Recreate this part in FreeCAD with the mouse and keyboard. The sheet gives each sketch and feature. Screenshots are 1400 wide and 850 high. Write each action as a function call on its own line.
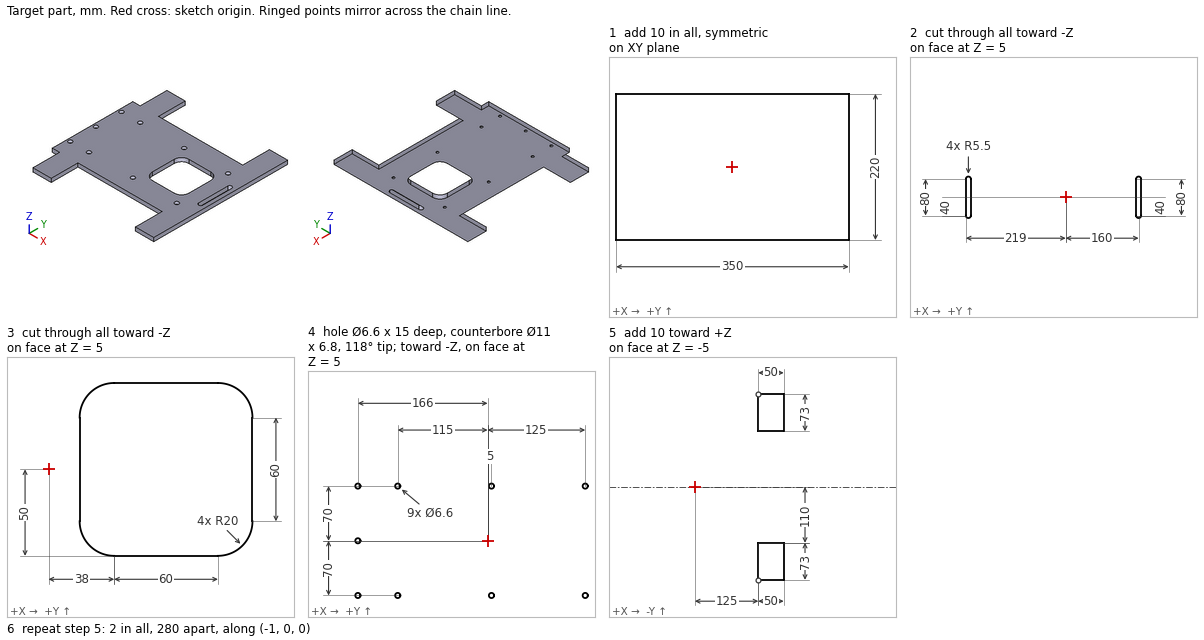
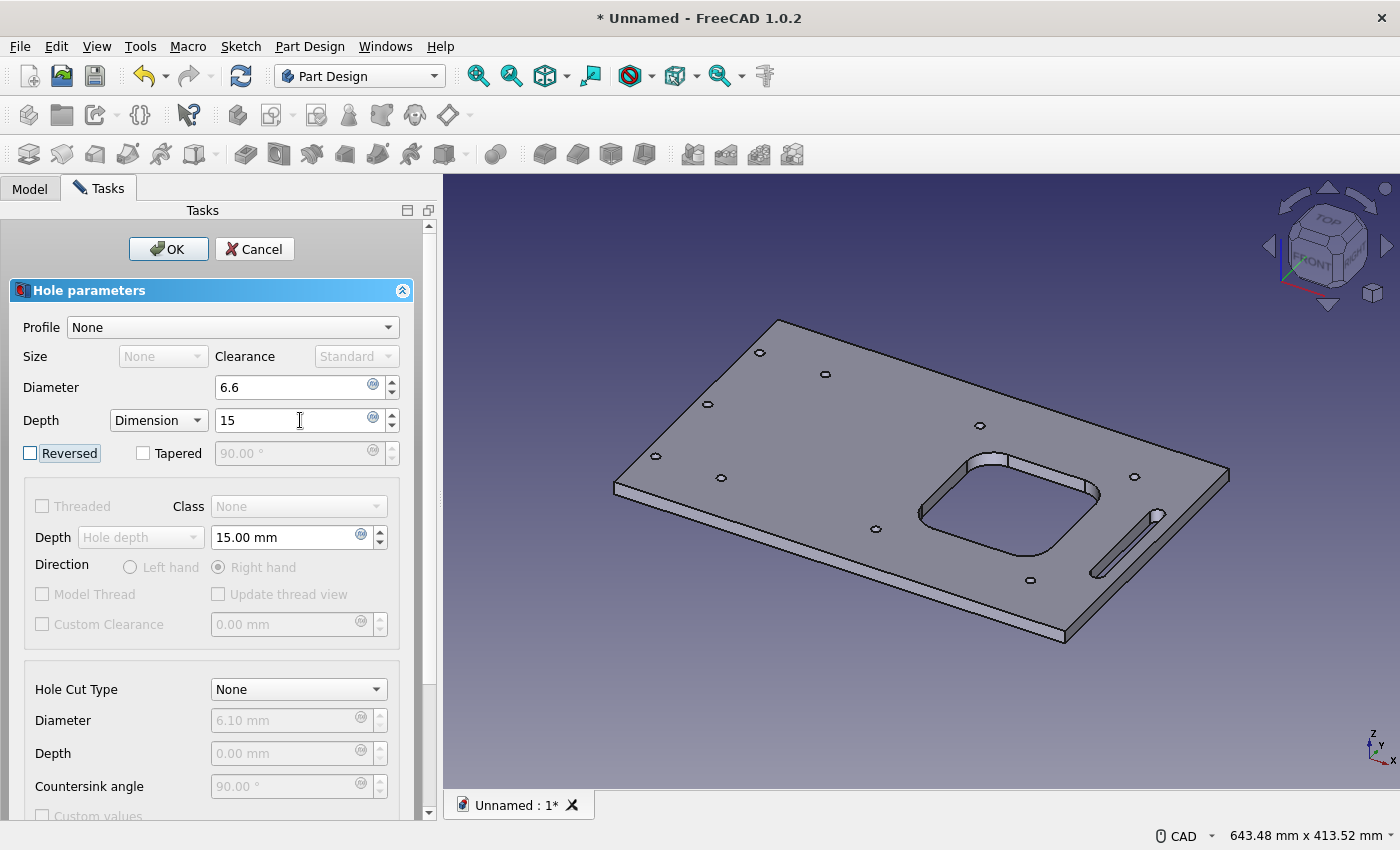
click(300, 690)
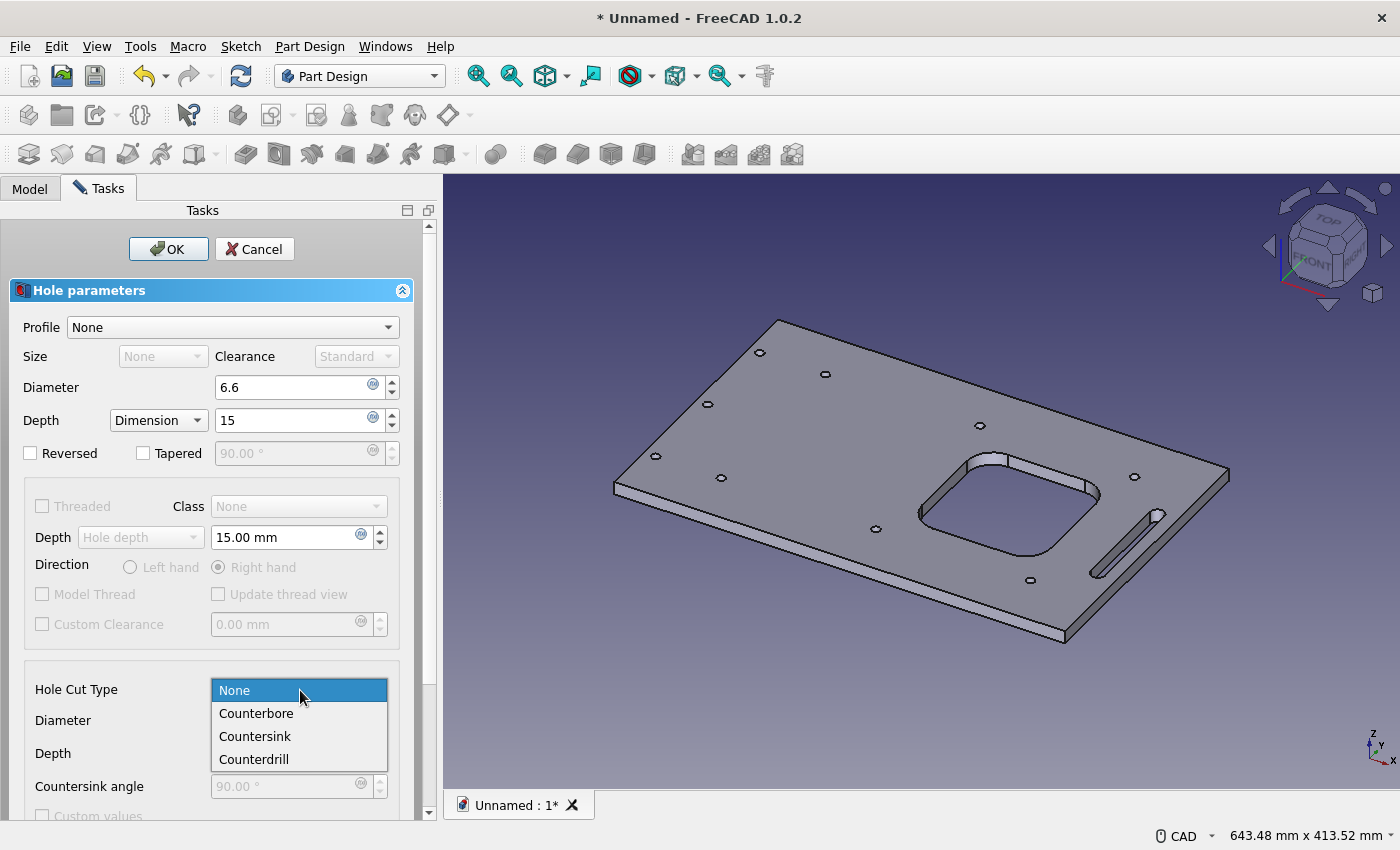
click(298, 714)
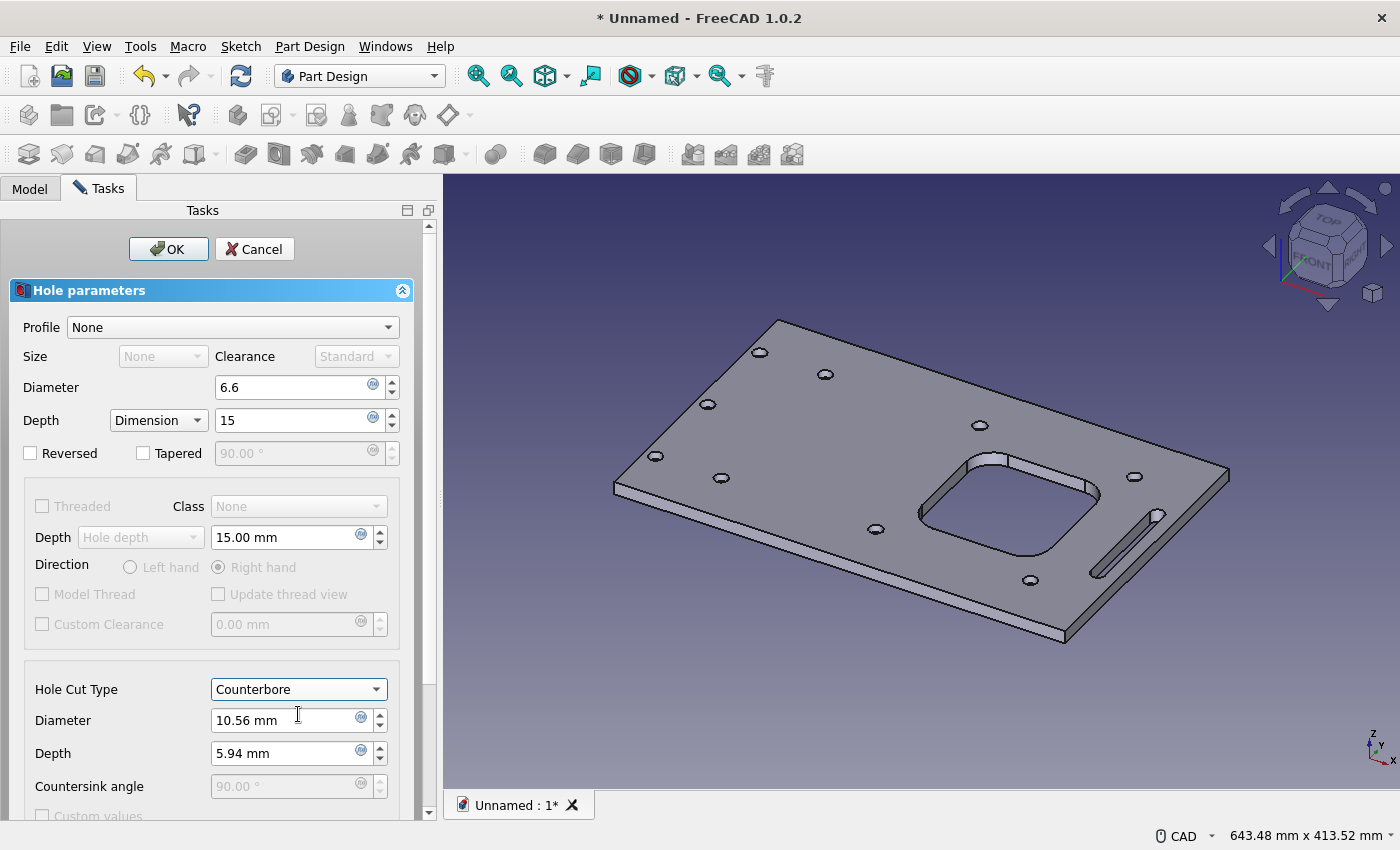
triple_click(292, 720)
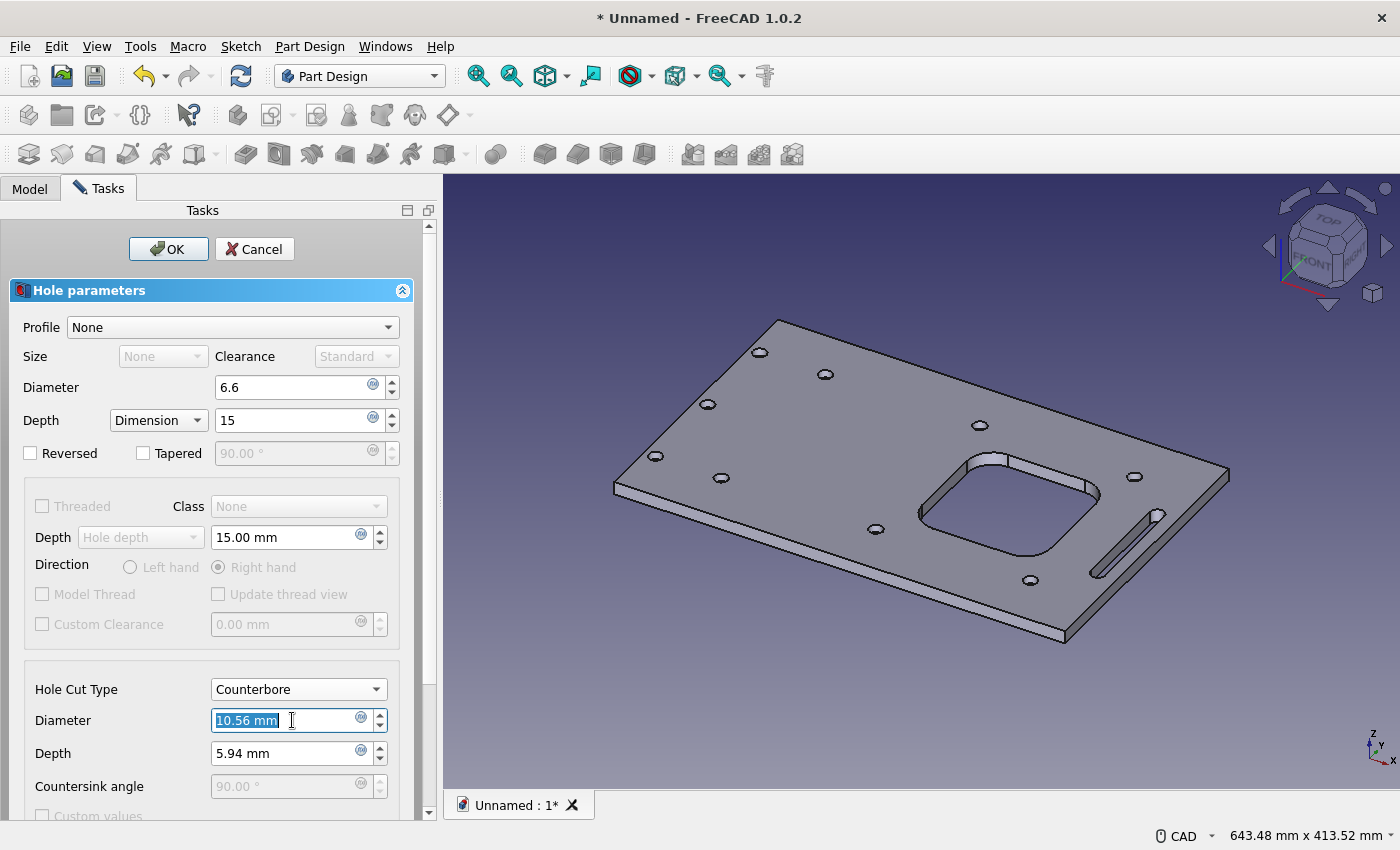
text(11)
key(Tab)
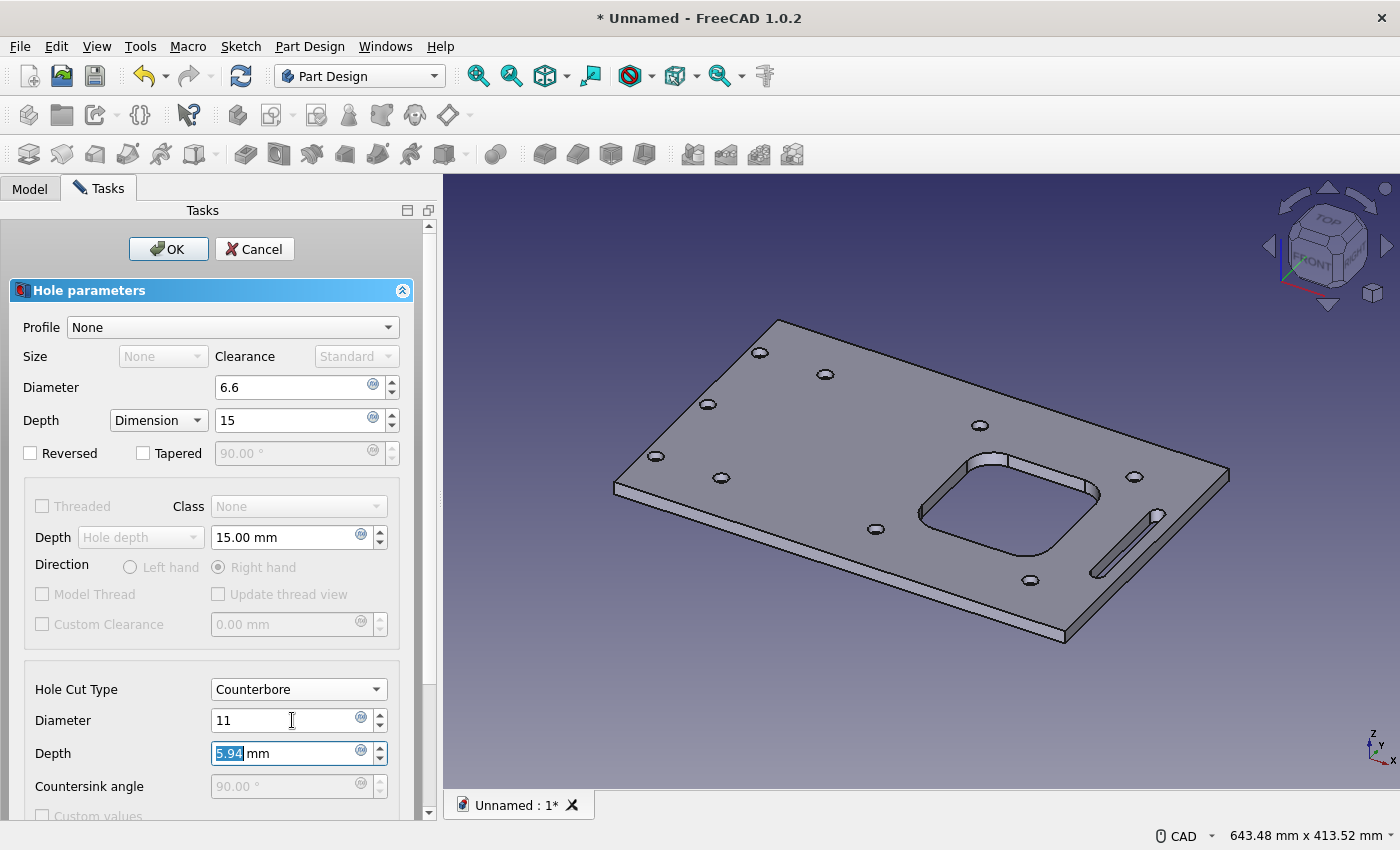
text(6.8)
key(Tab)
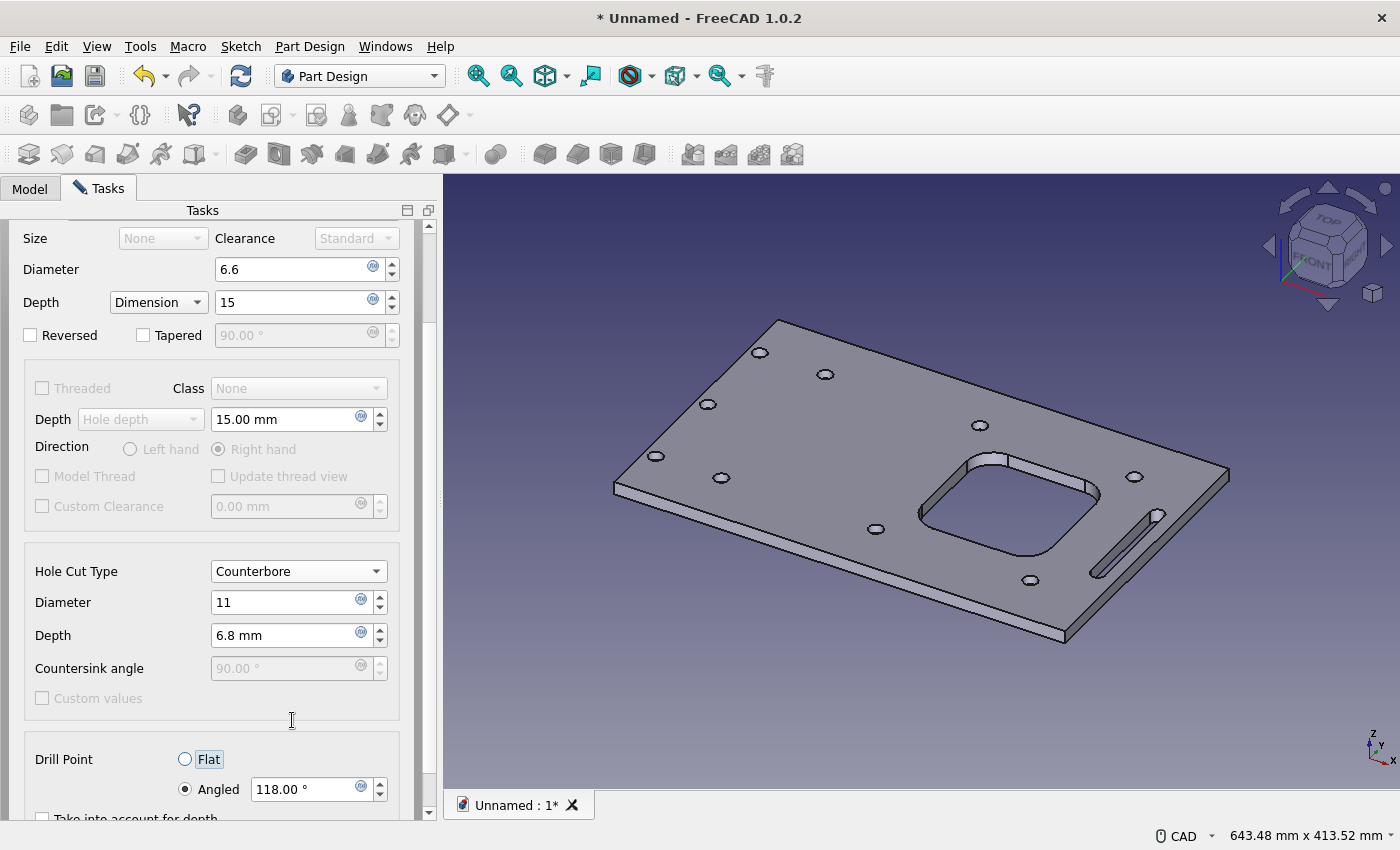
scroll(429, 520, up, 3)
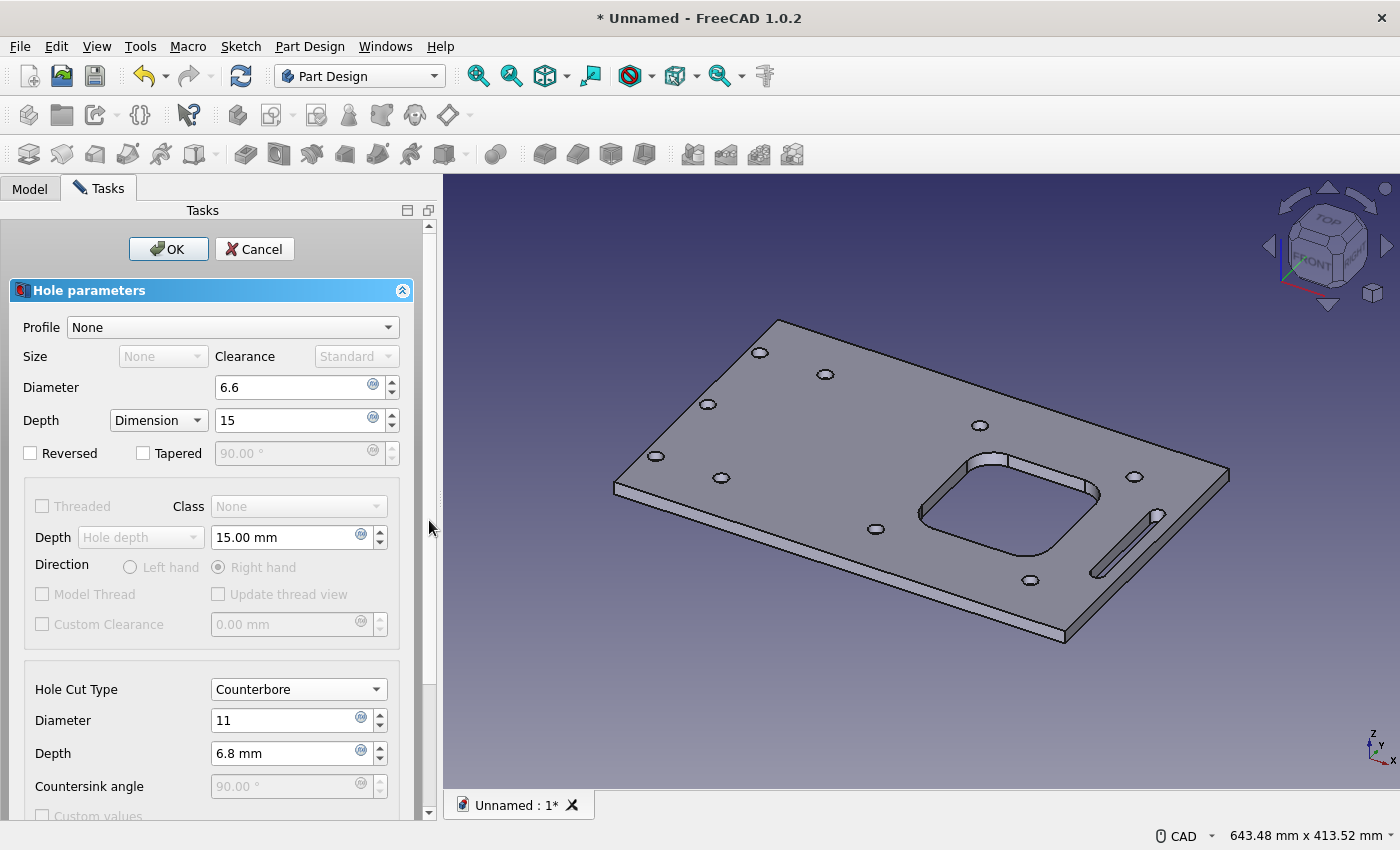
click(169, 249)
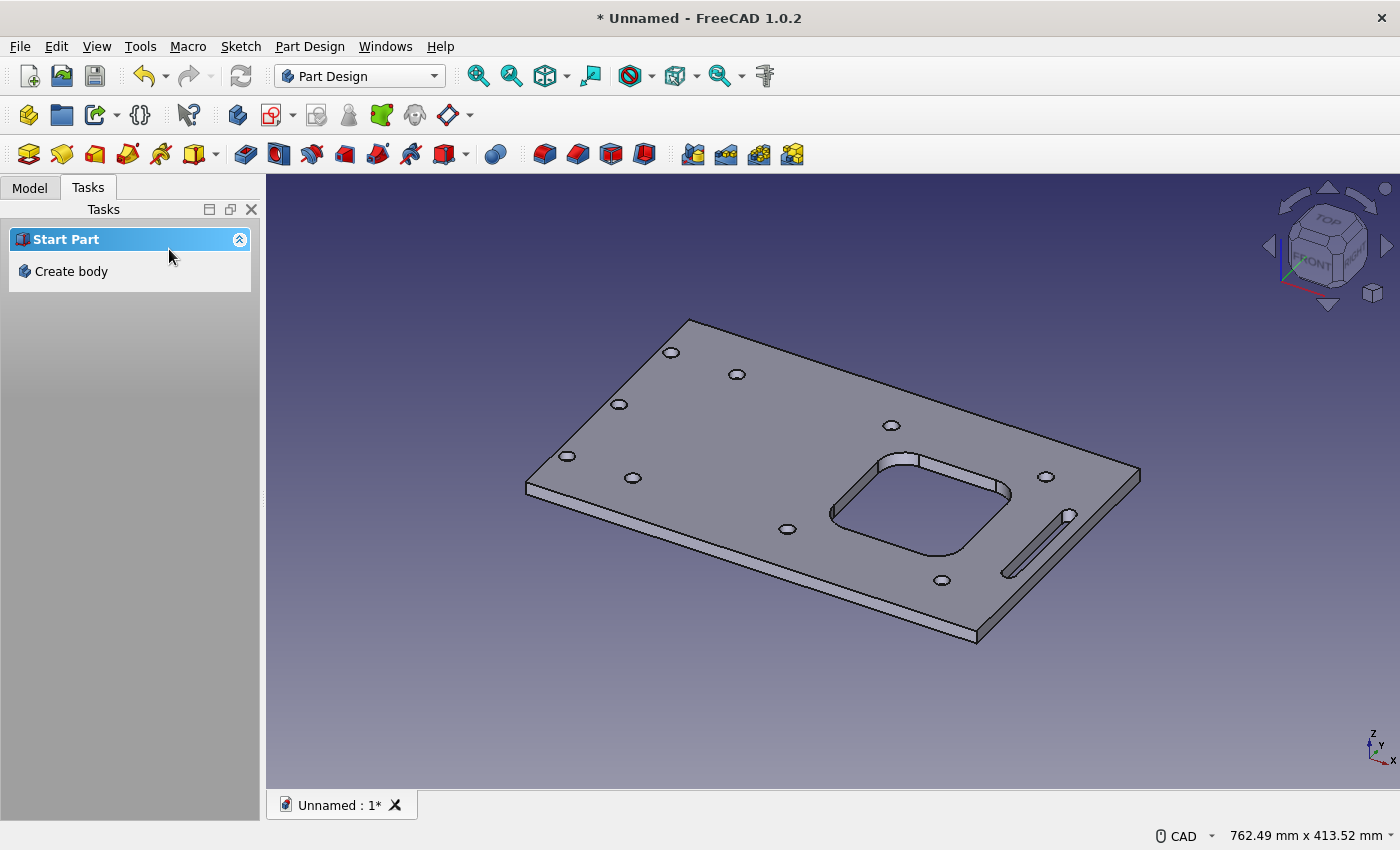
key(5)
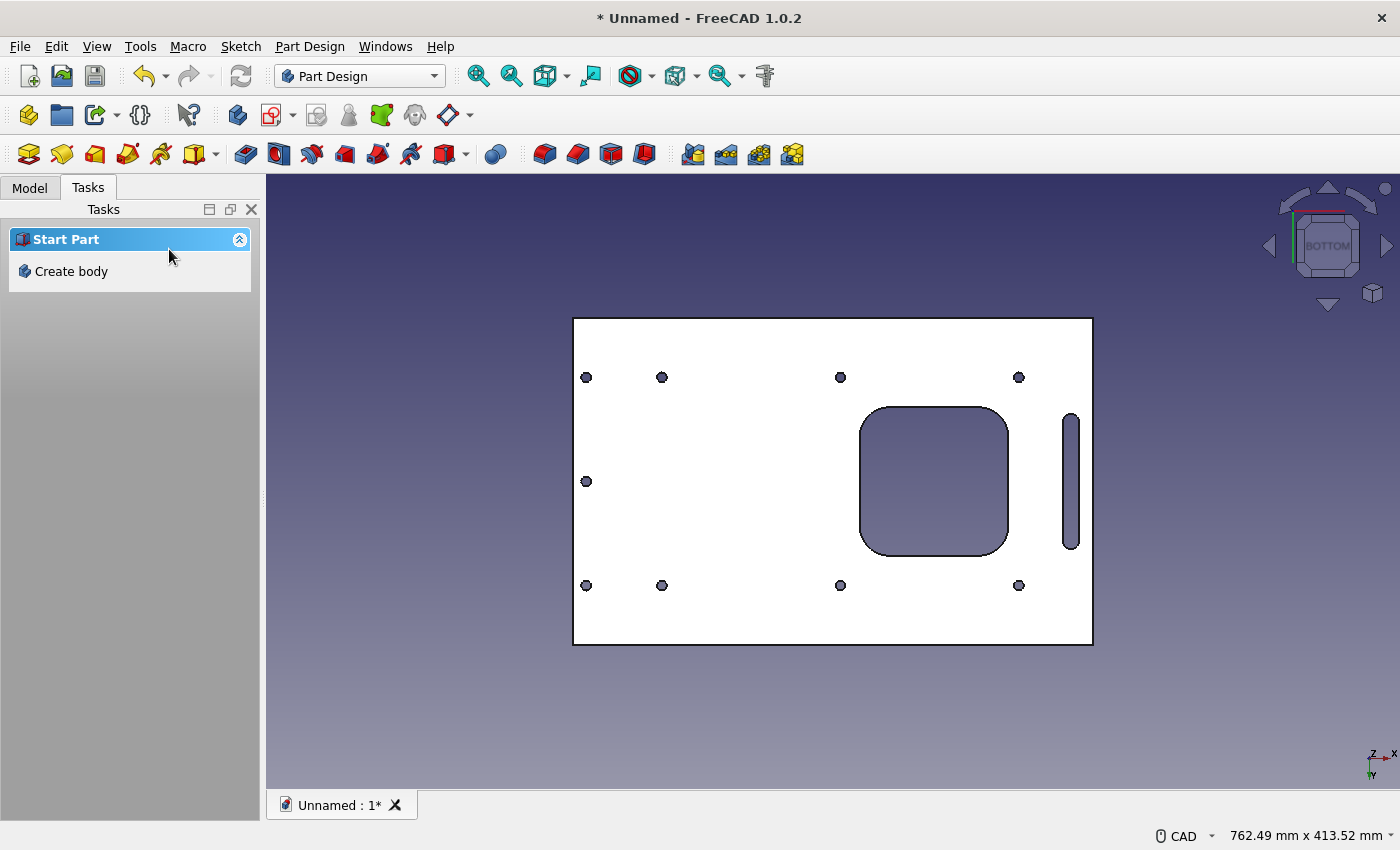
click(759, 480)